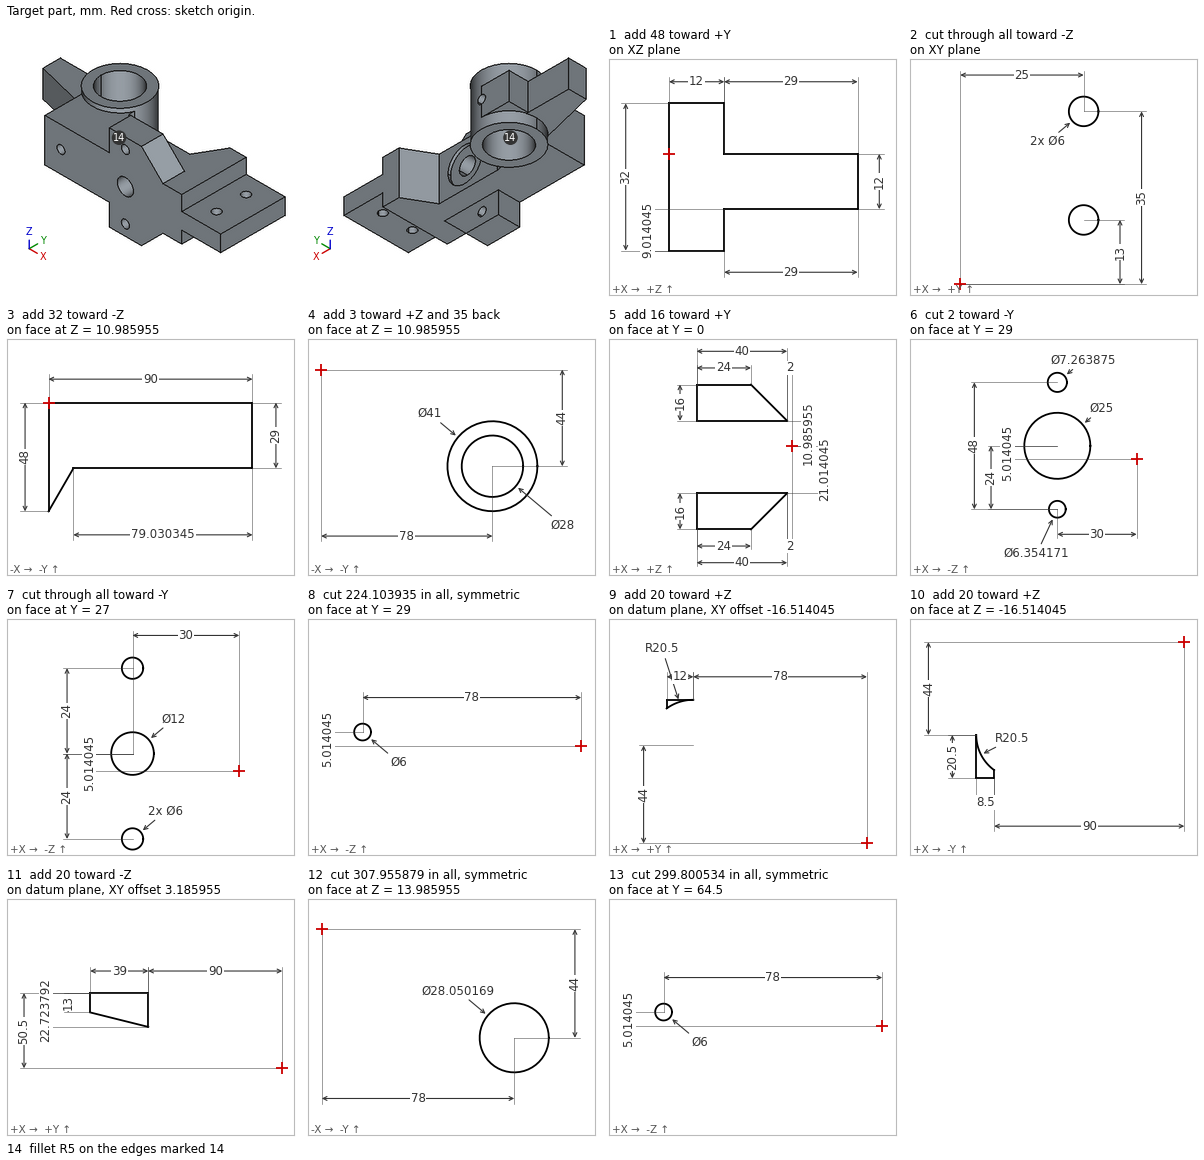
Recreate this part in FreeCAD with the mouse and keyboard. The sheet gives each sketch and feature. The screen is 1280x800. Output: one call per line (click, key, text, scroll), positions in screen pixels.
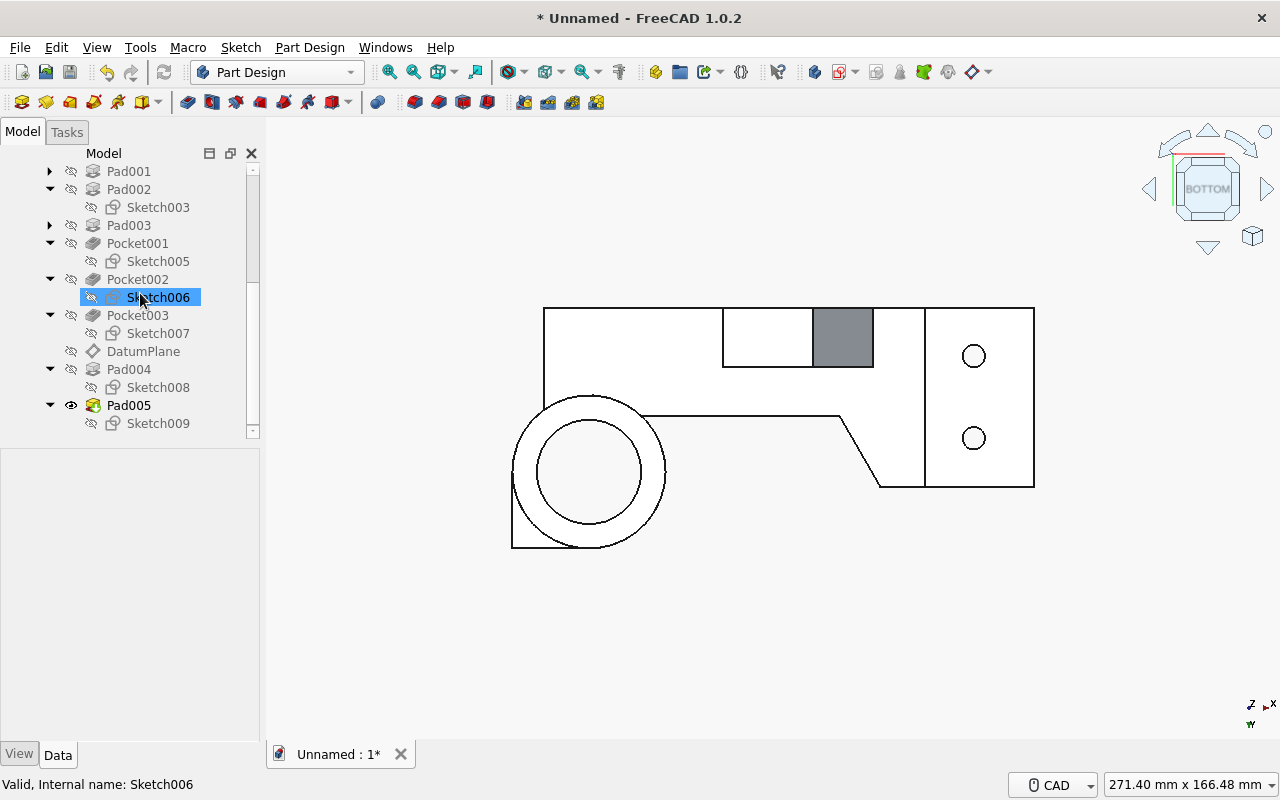
scroll(140, 293, up, 15)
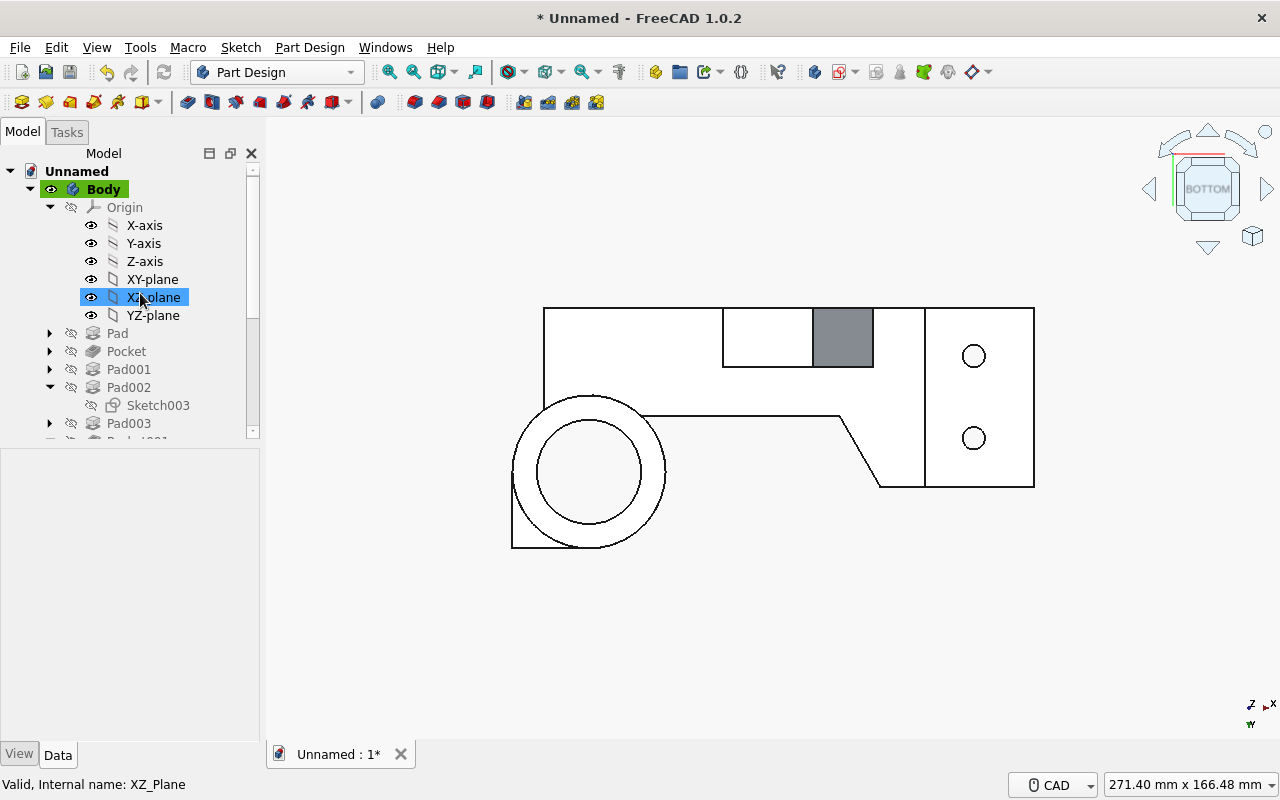
click(136, 279)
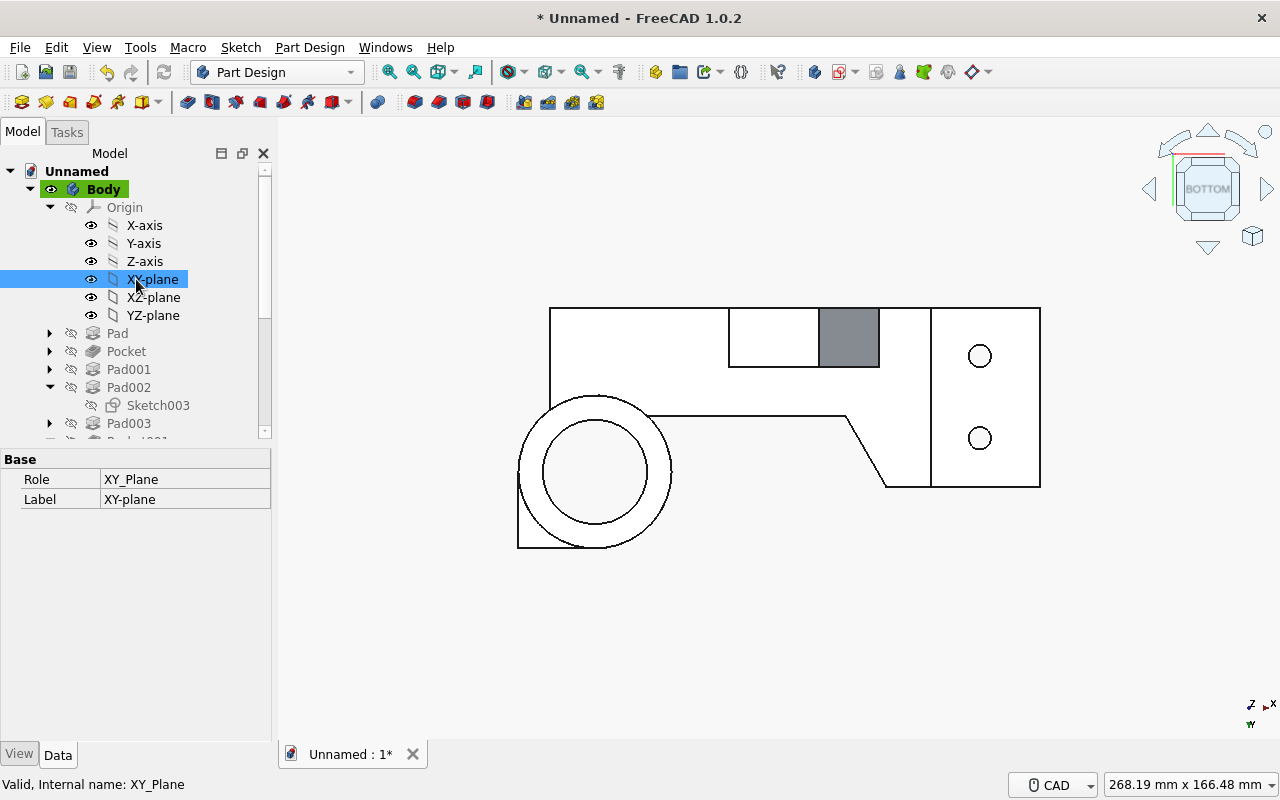
click(972, 72)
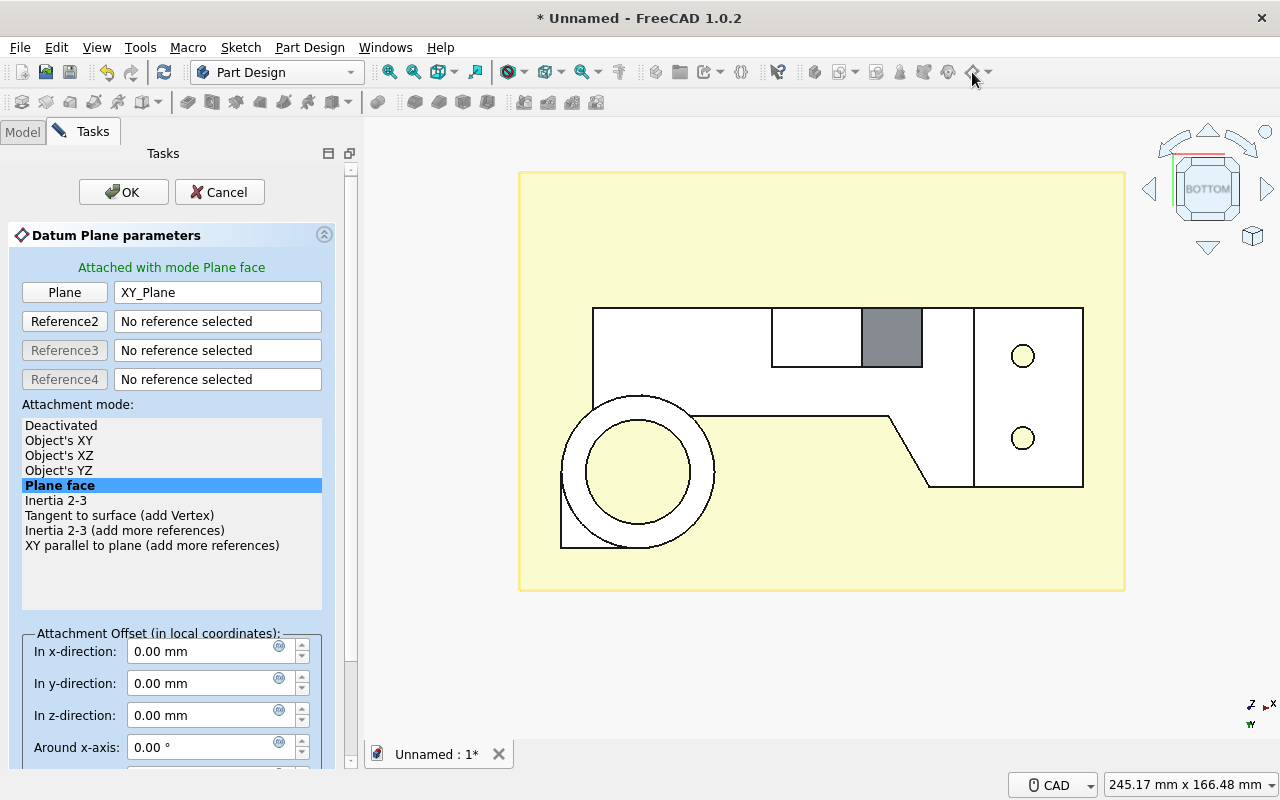
triple_click(210, 715)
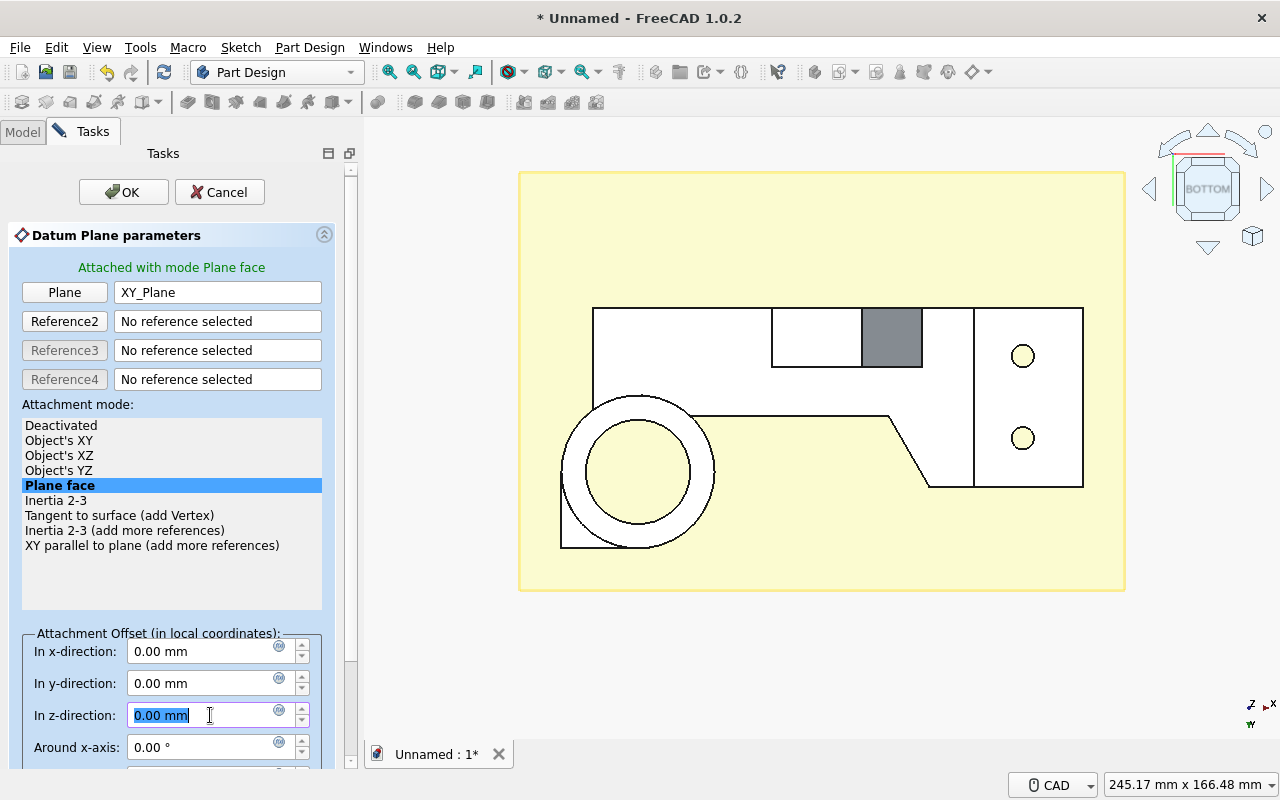
text(3.185955)
key(Tab)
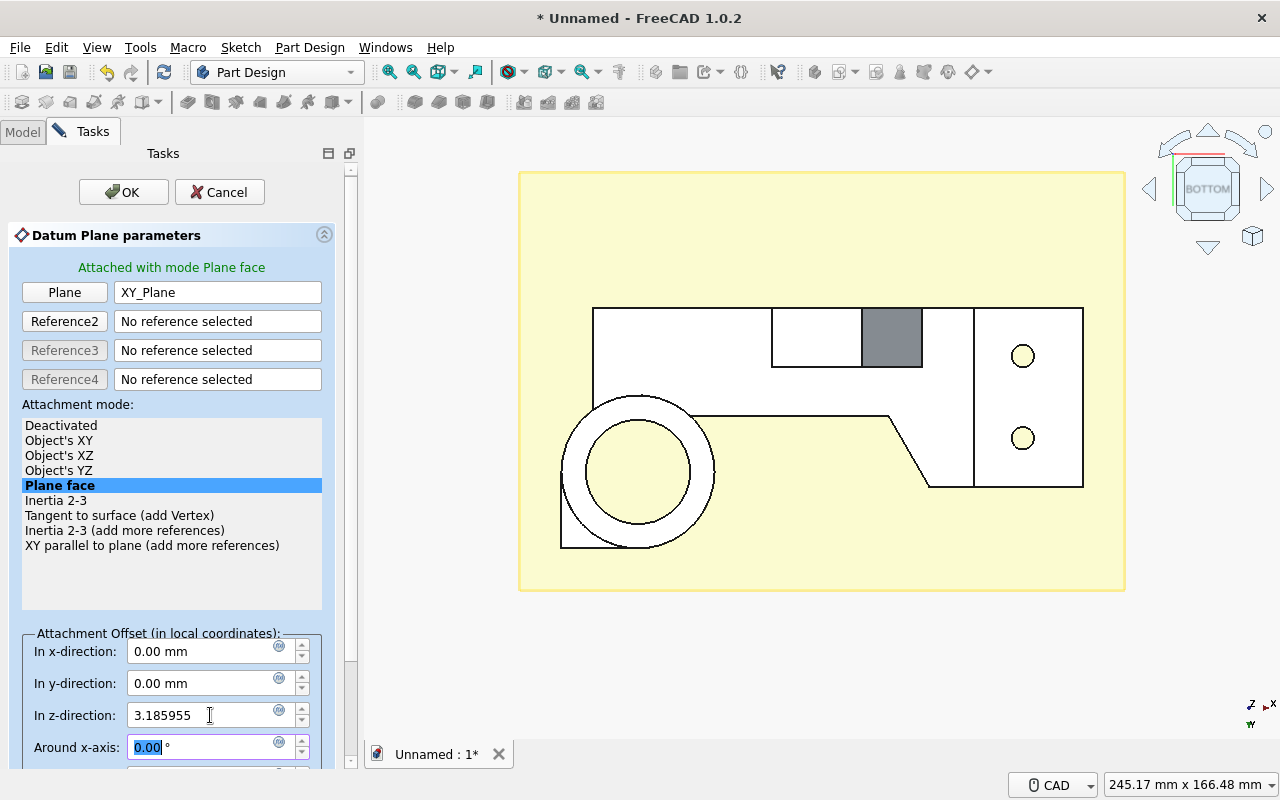
click(124, 192)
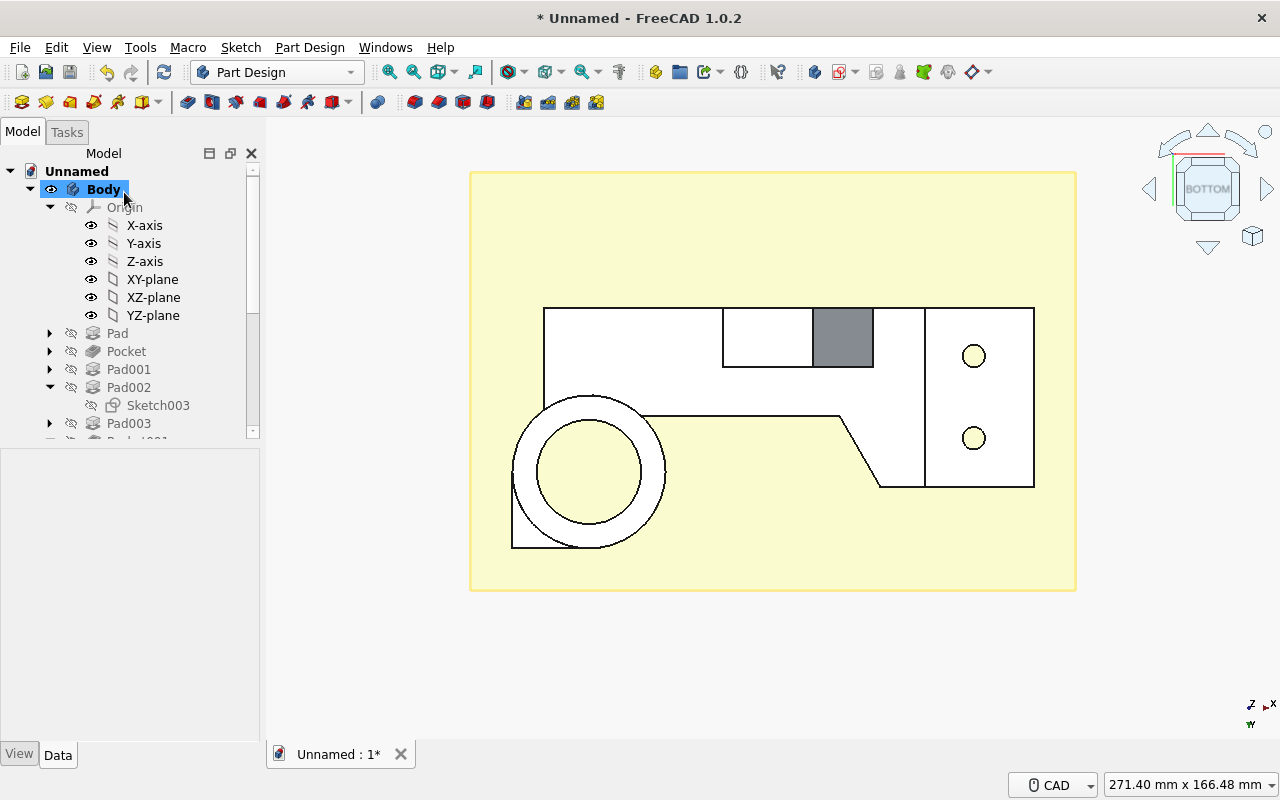
scroll(100, 293, down, 3)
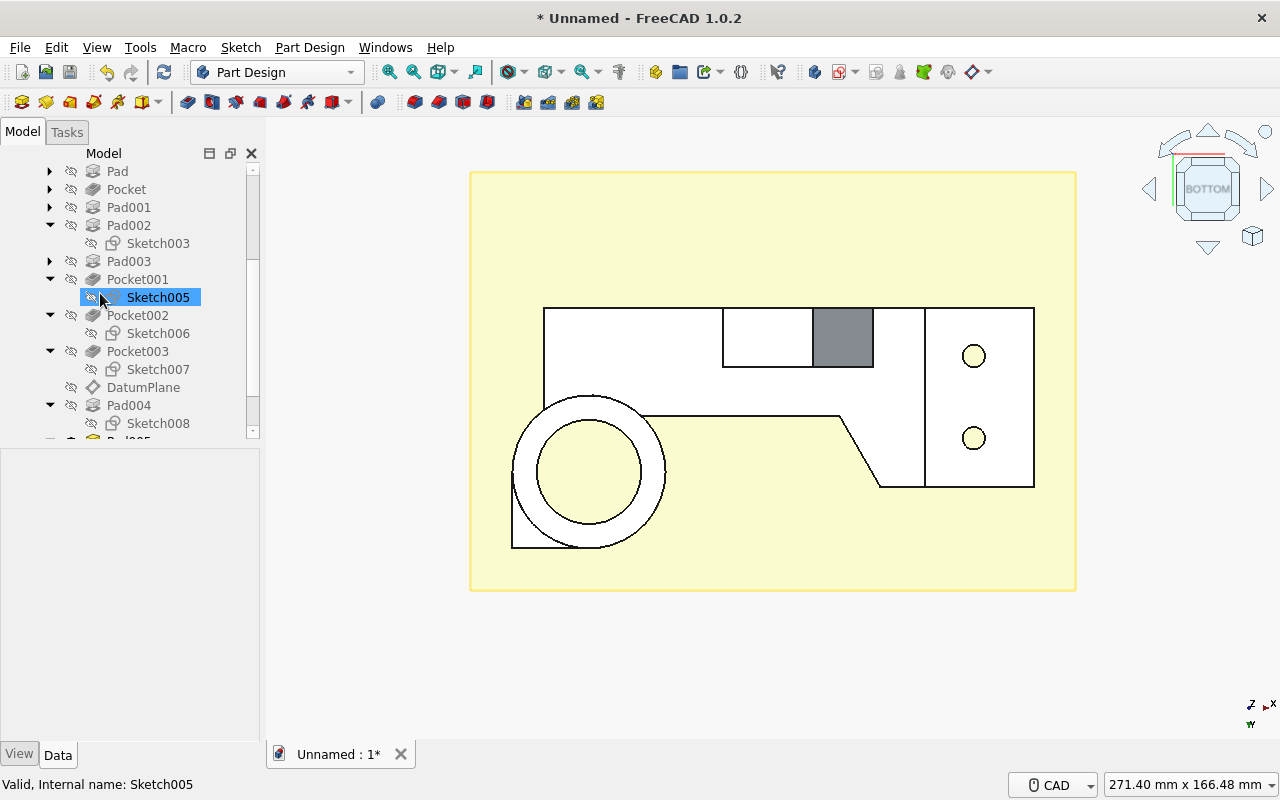
scroll(140, 293, up, 15)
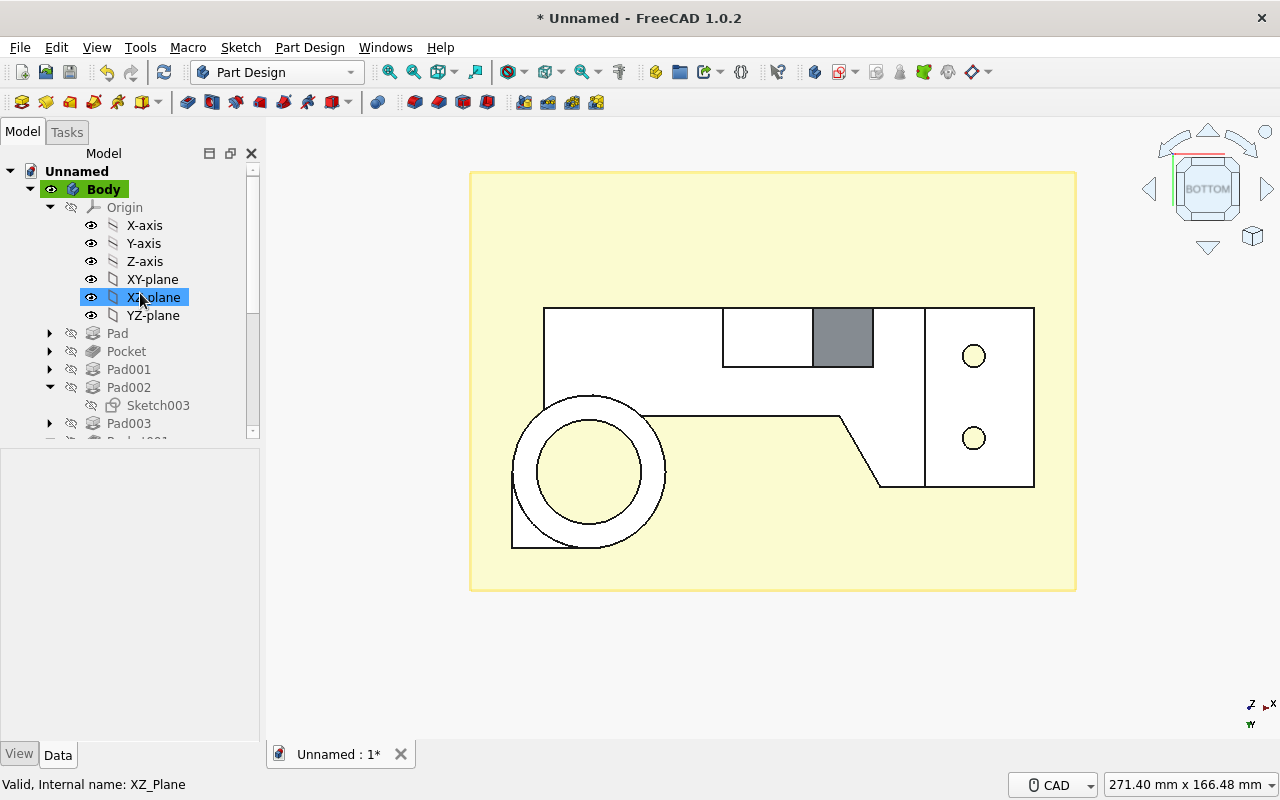
scroll(100, 293, down, 6)